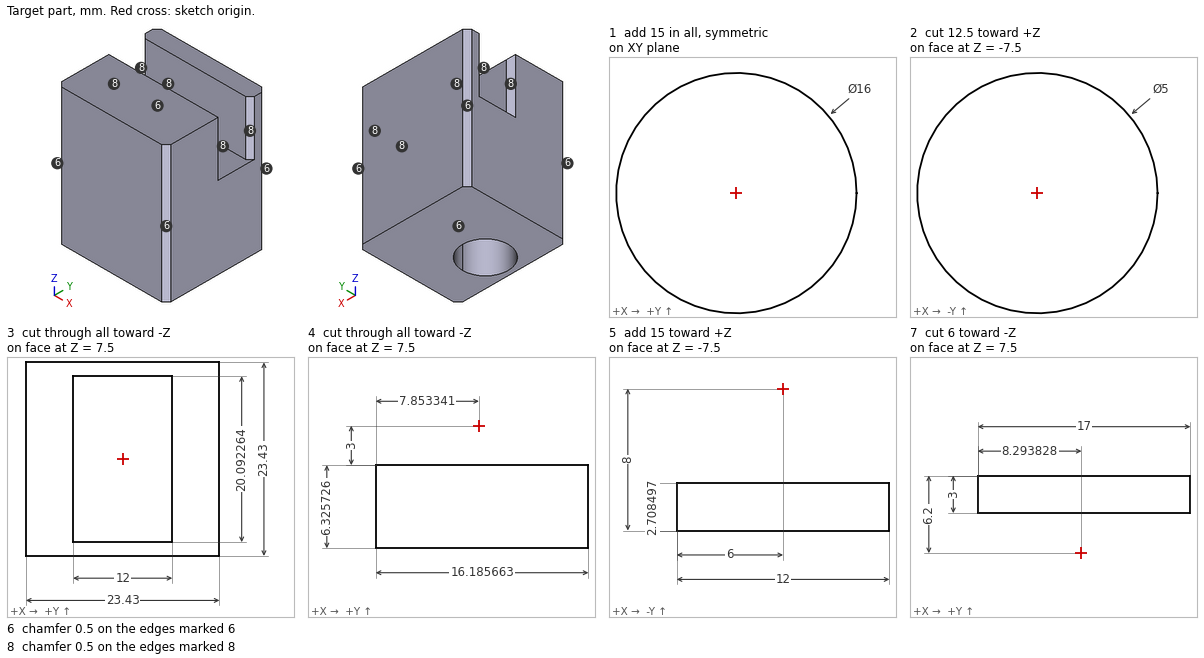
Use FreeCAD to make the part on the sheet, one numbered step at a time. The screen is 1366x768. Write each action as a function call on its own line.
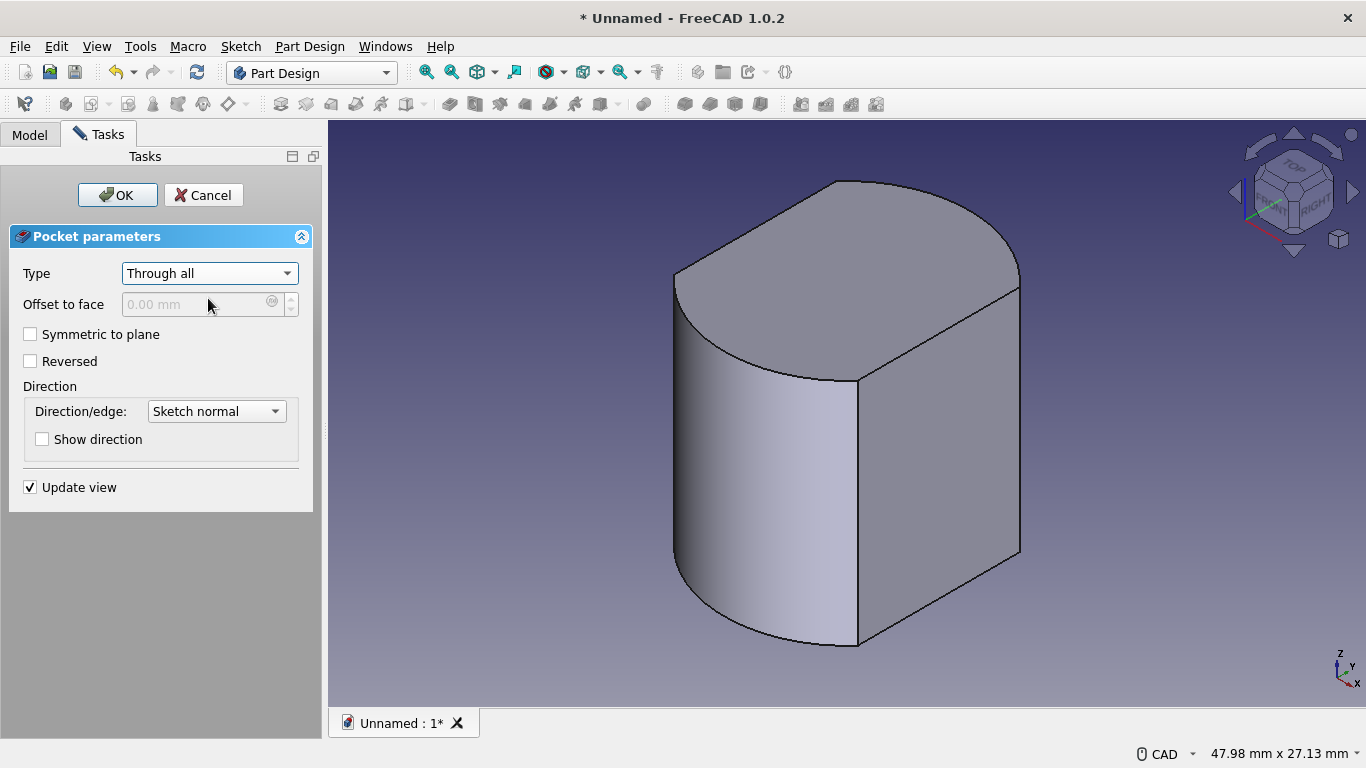
click(118, 195)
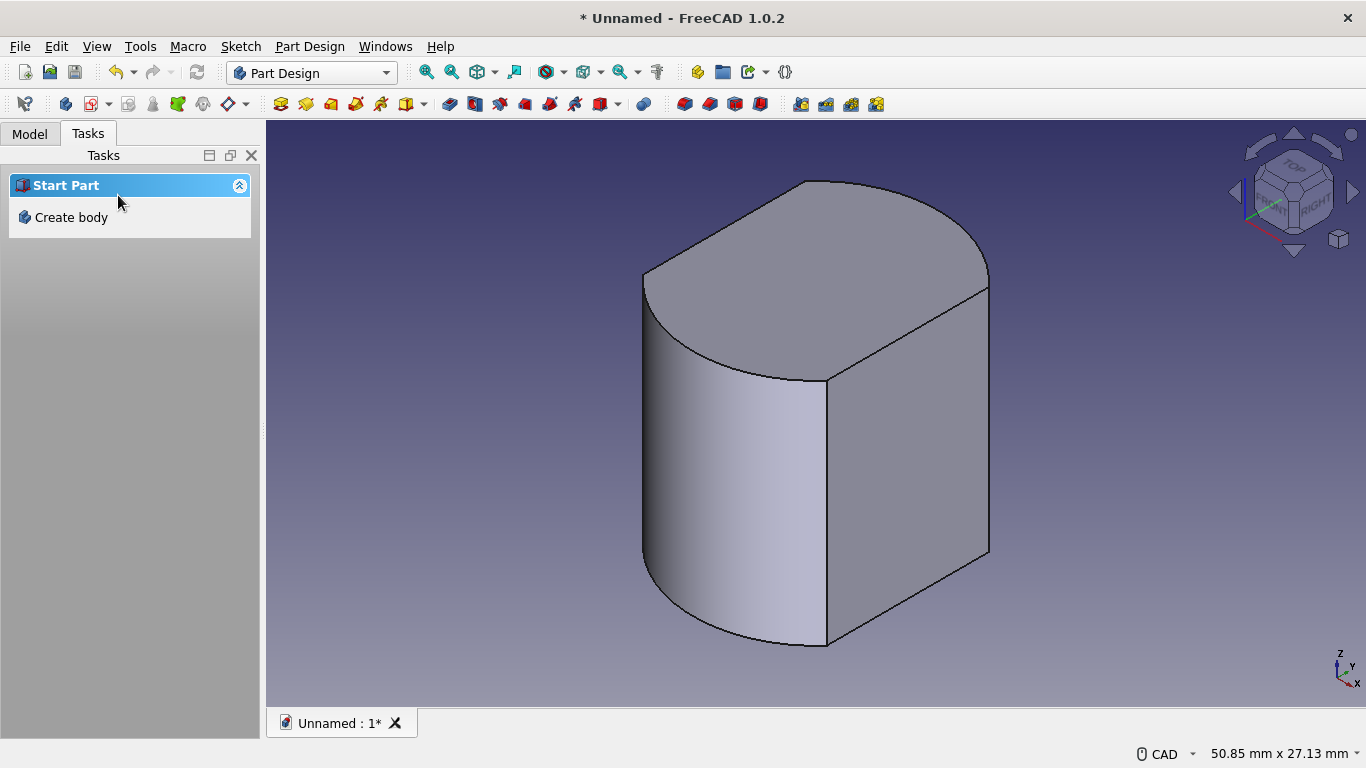
click(816, 280)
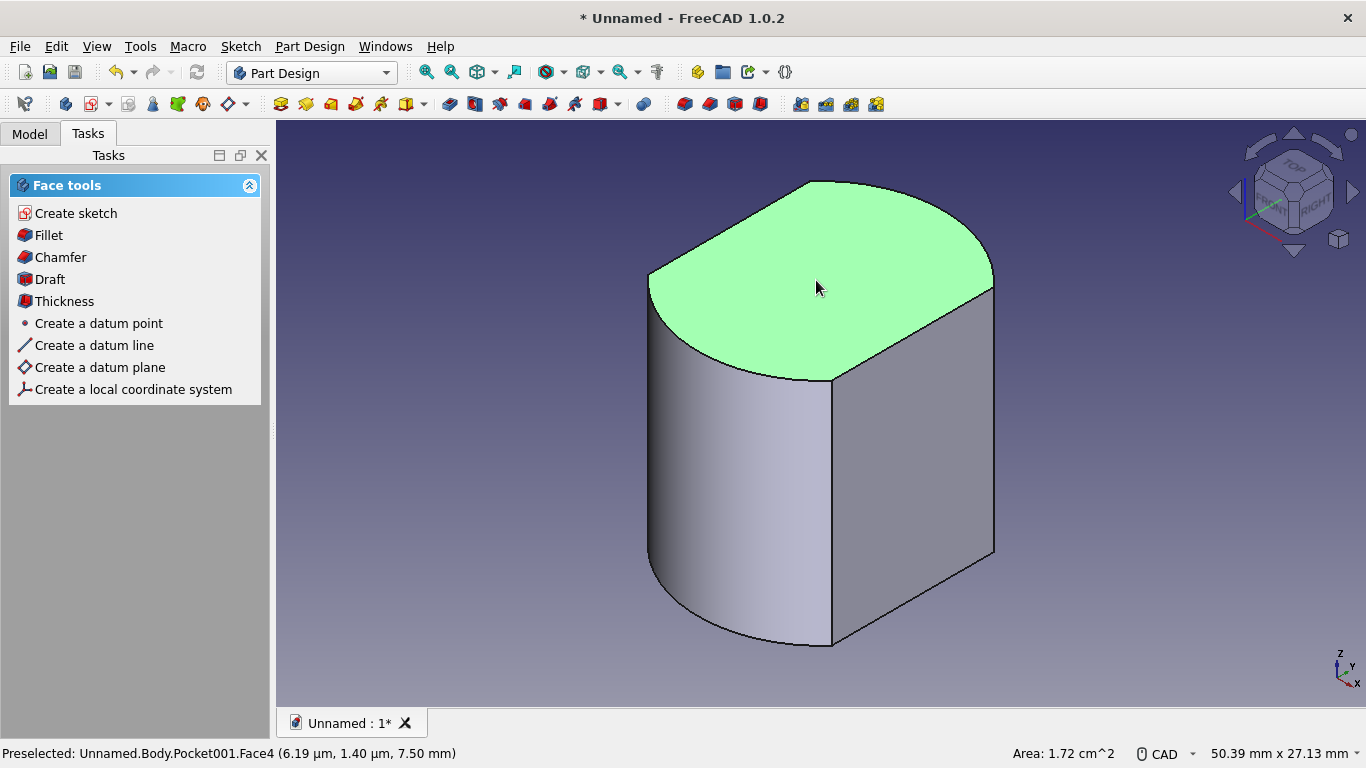
click(90, 104)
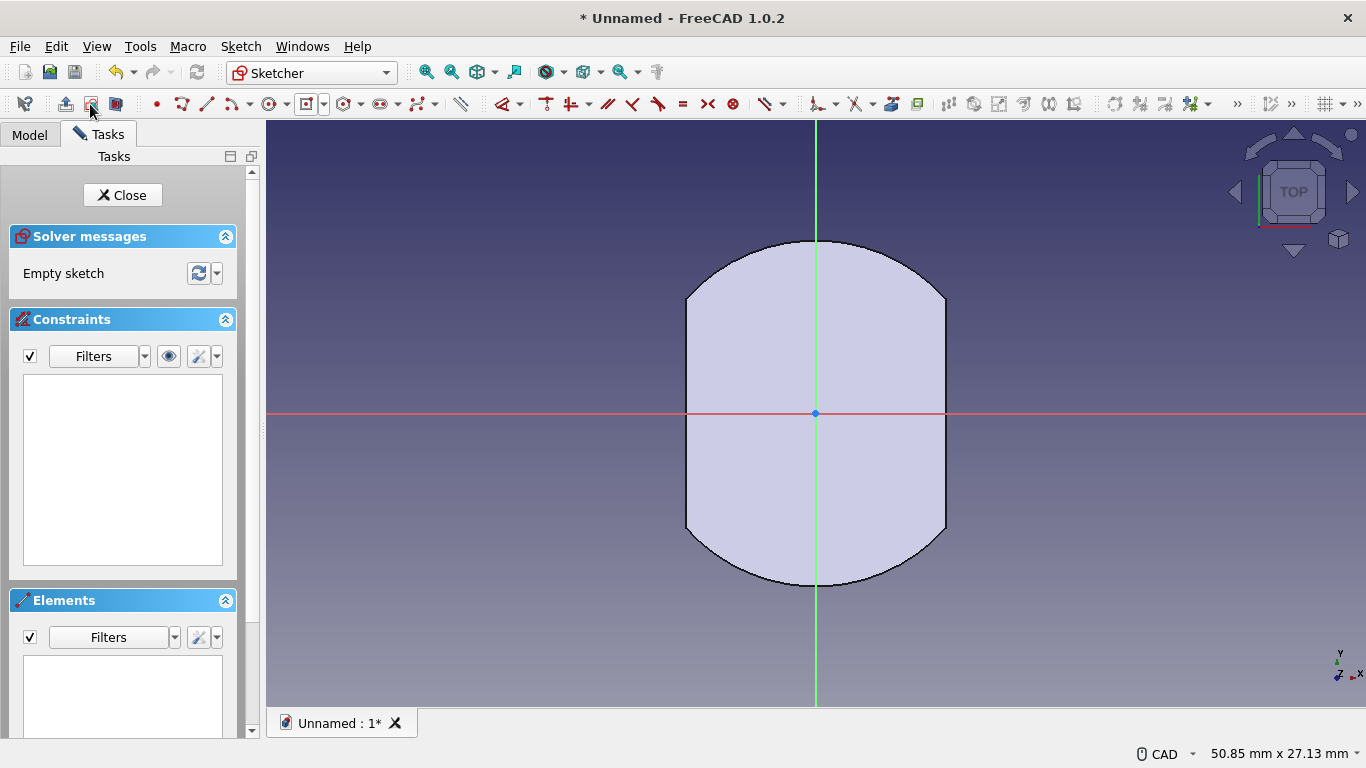
scroll(911, 637, up, 3)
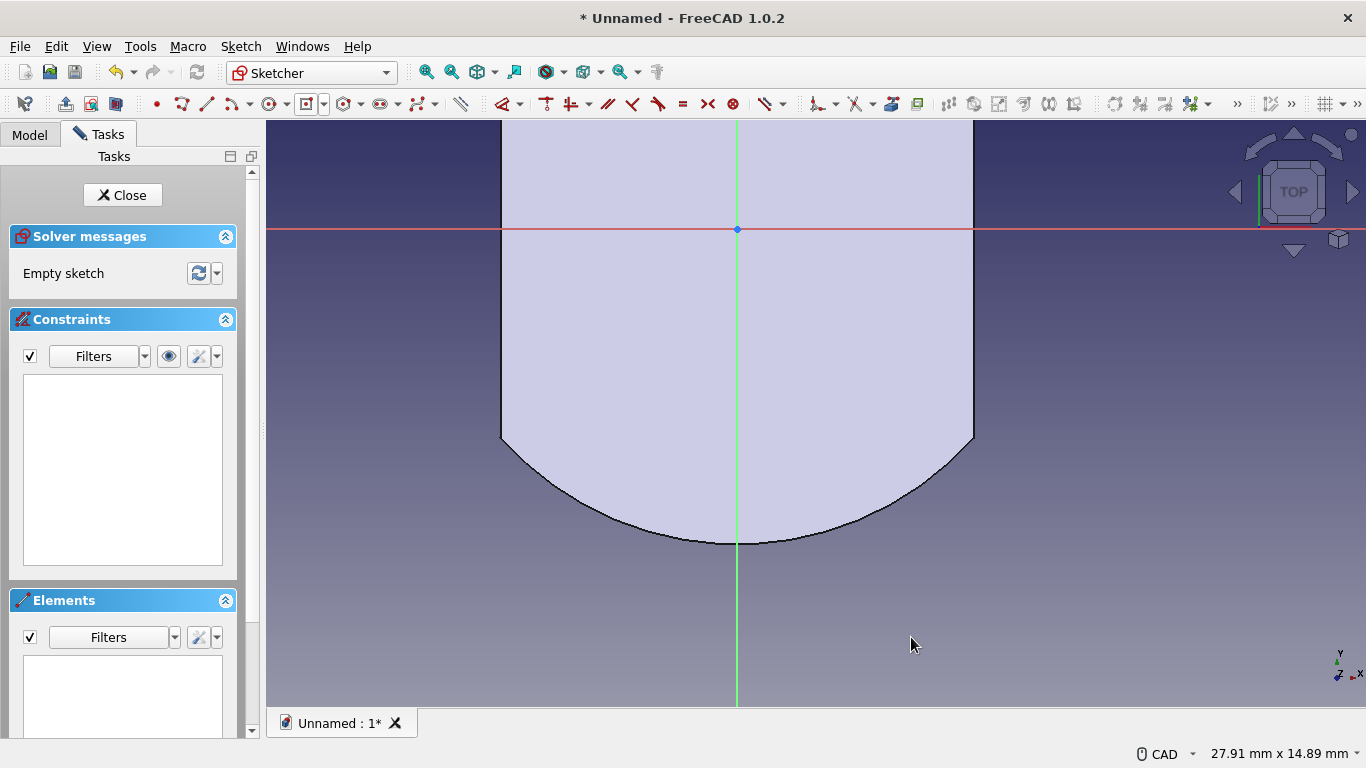
key(g)
key(r)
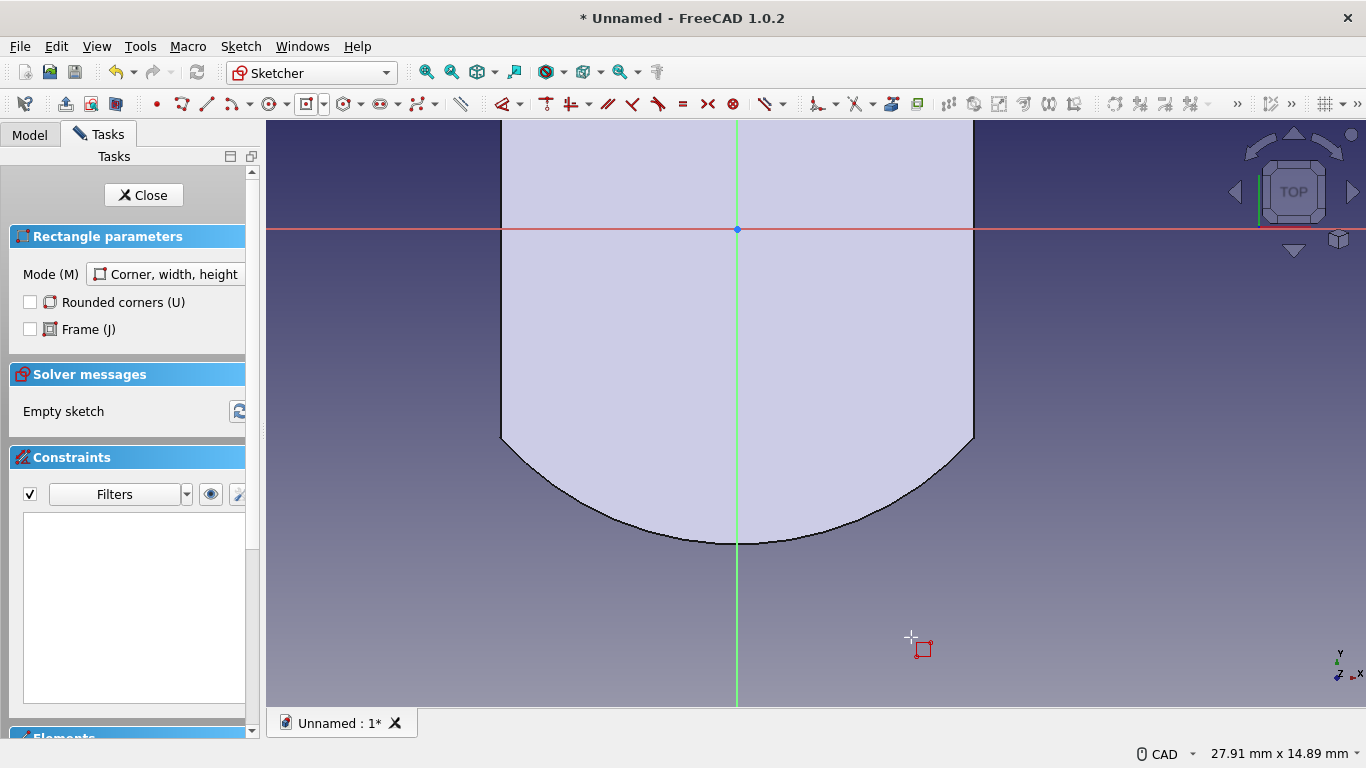
click(428, 347)
click(1066, 597)
key(Escape)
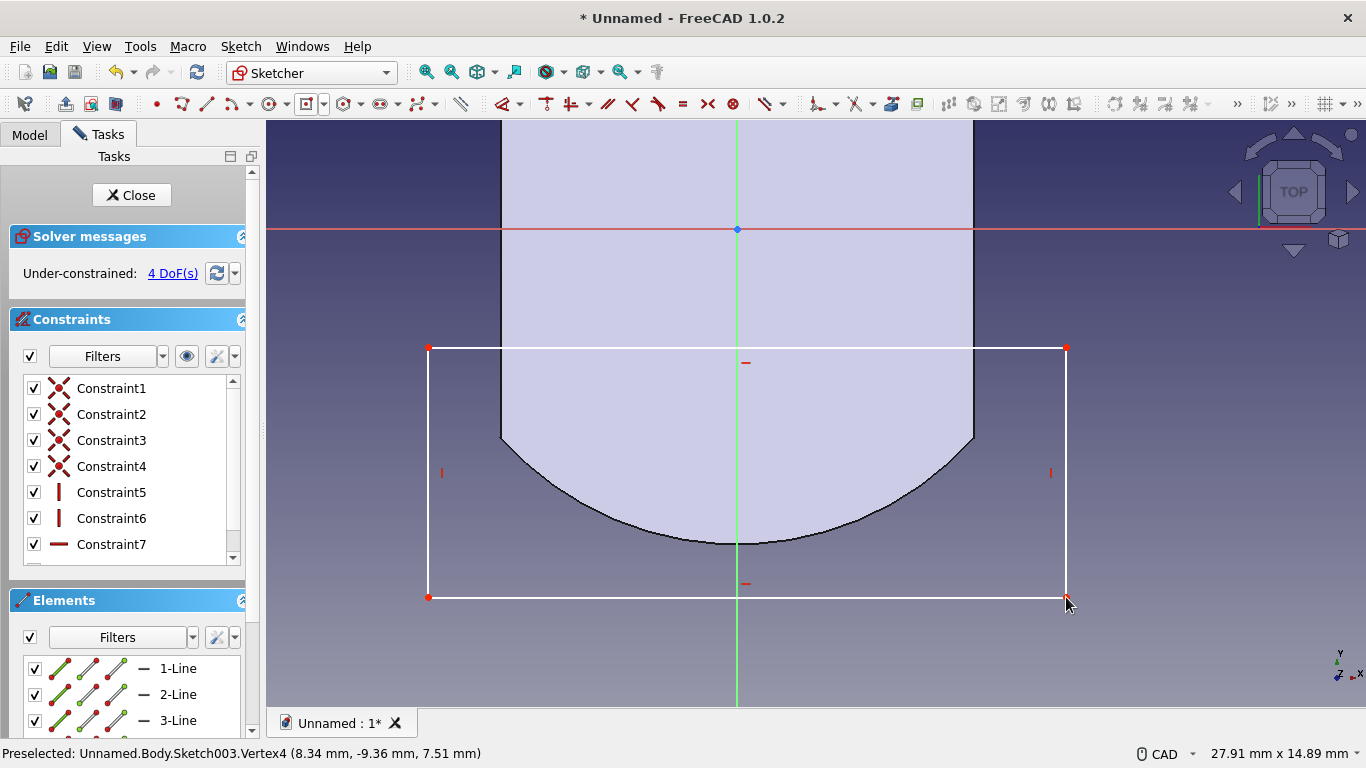
click(502, 104)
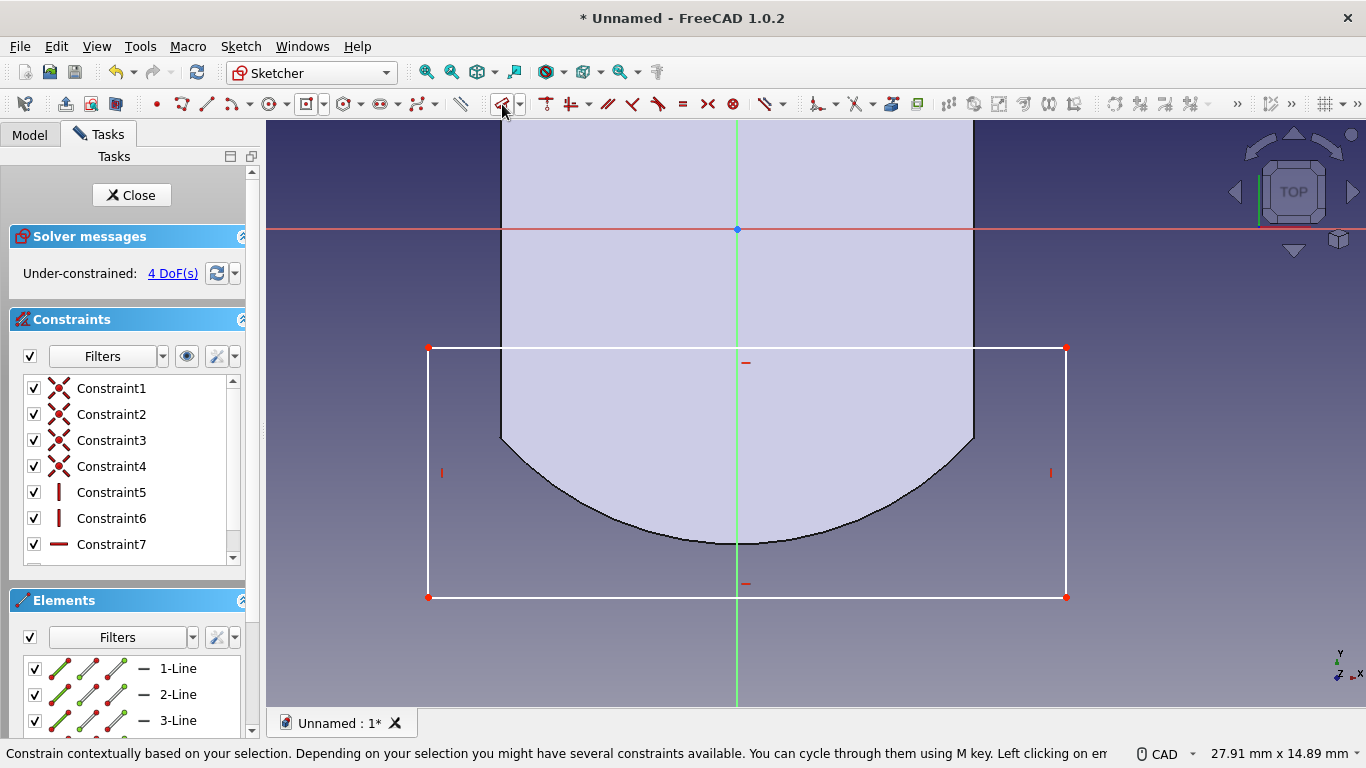
click(428, 348)
click(394, 289)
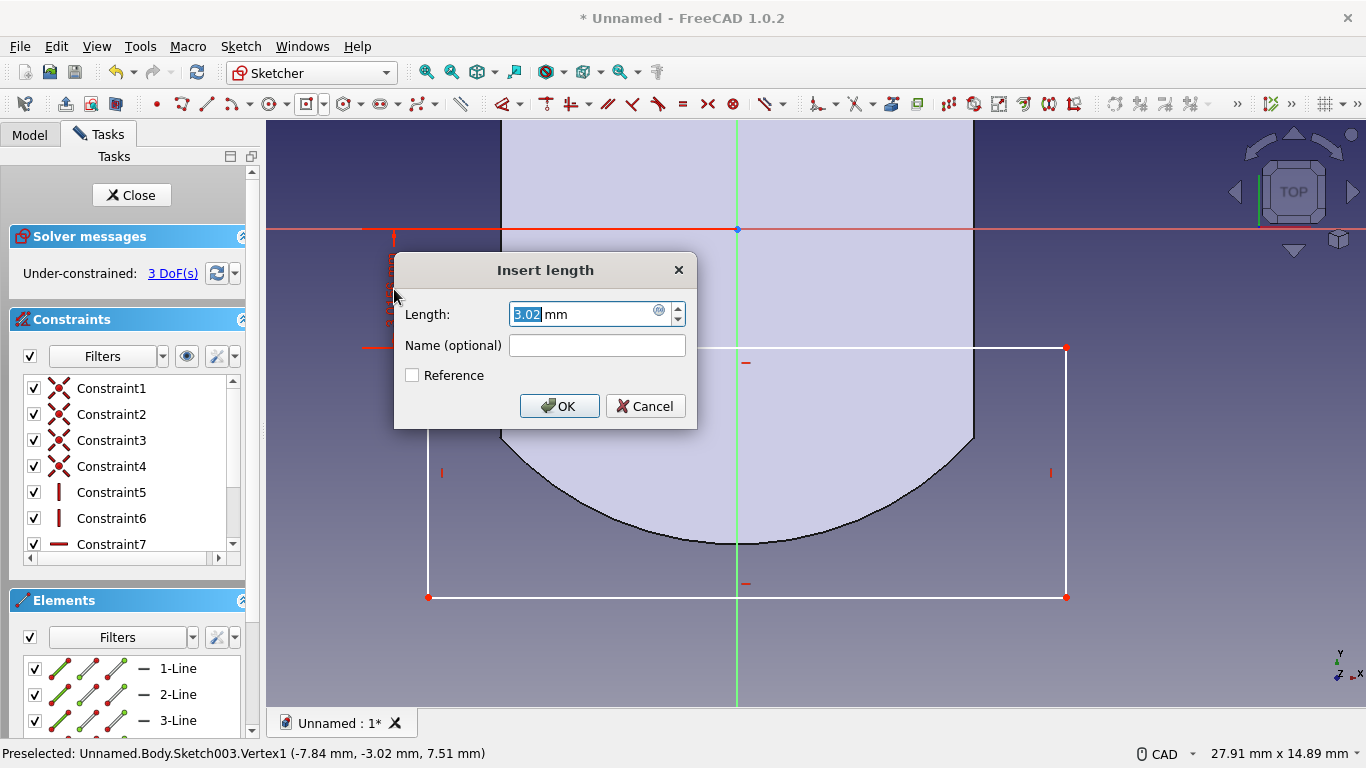
text(3)
key(Return)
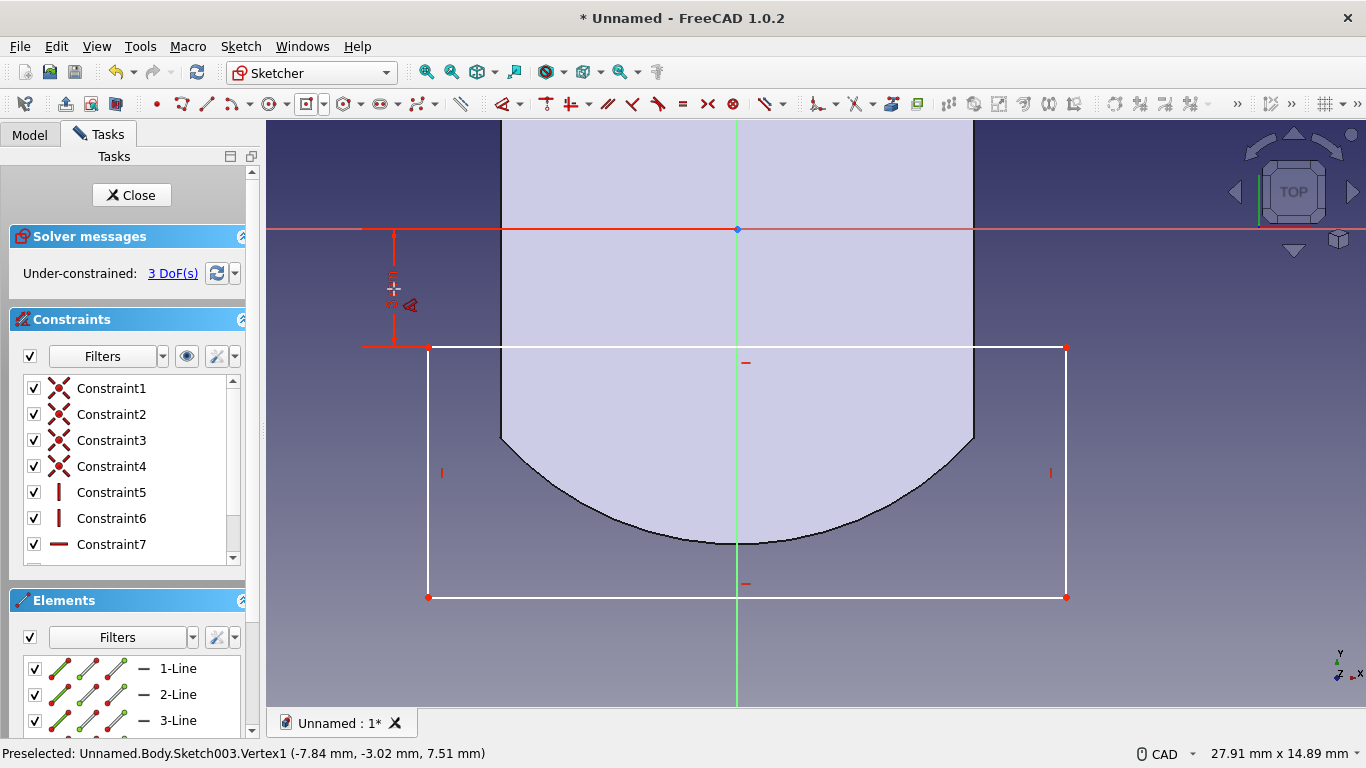
click(428, 423)
click(394, 473)